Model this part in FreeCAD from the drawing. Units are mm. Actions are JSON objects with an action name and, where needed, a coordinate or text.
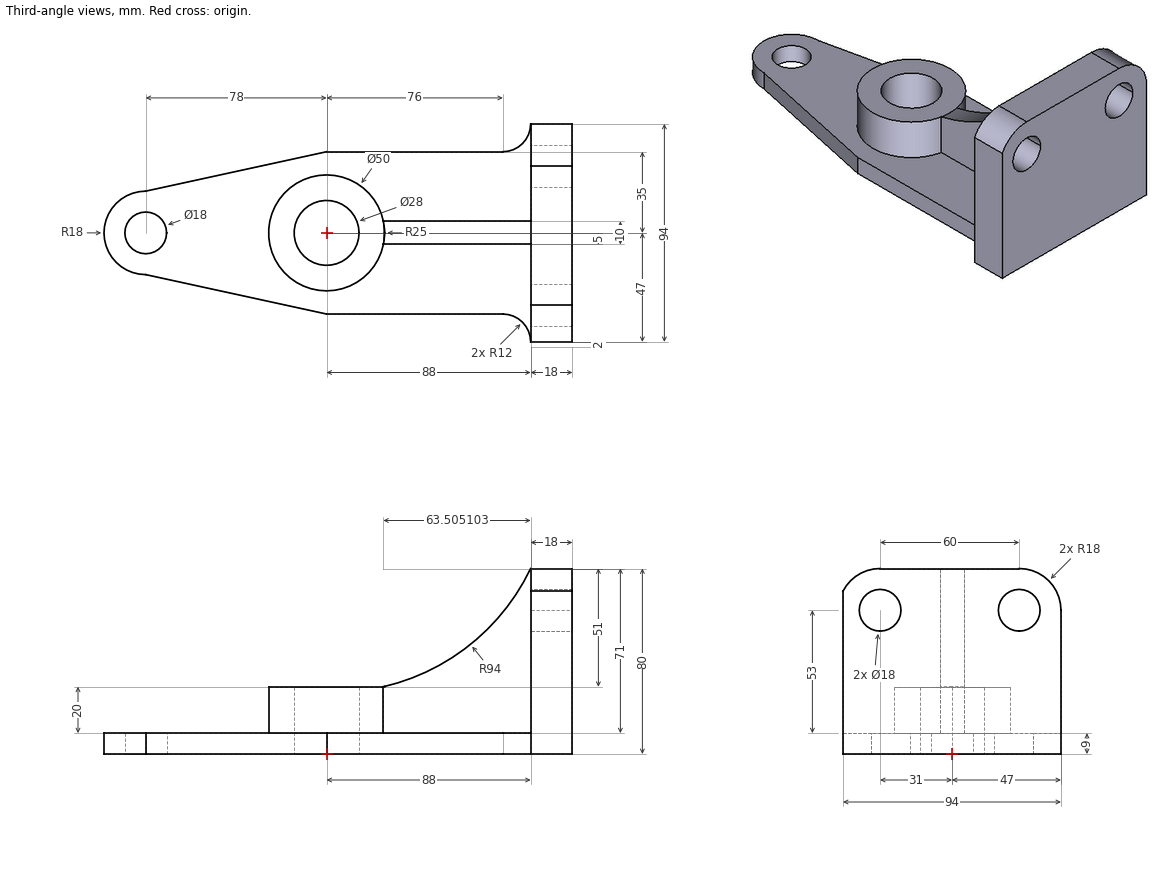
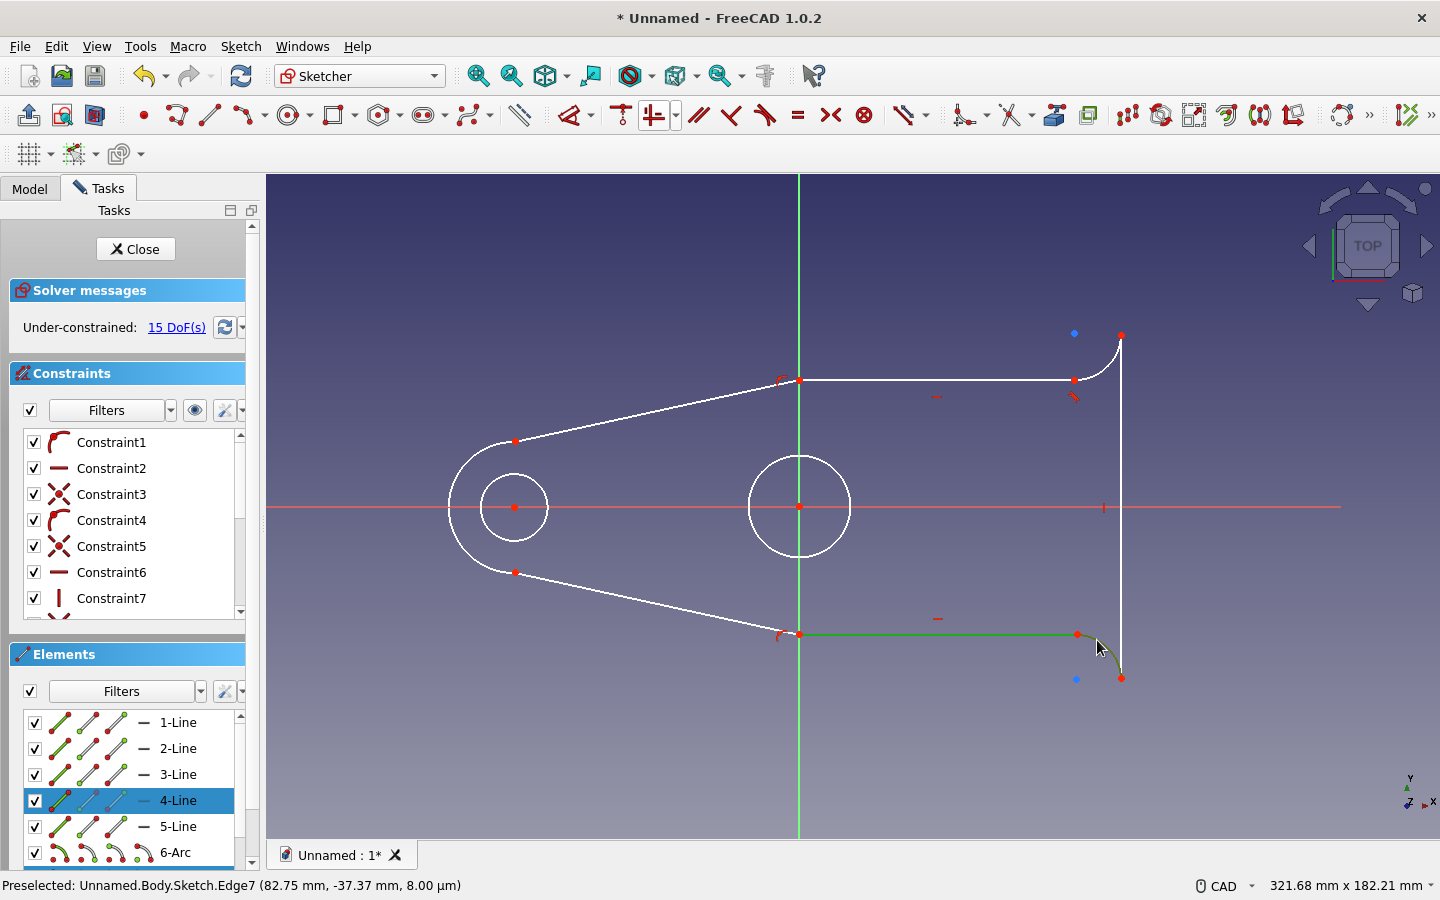
{"action": "left_click", "coordinate": [765, 116]}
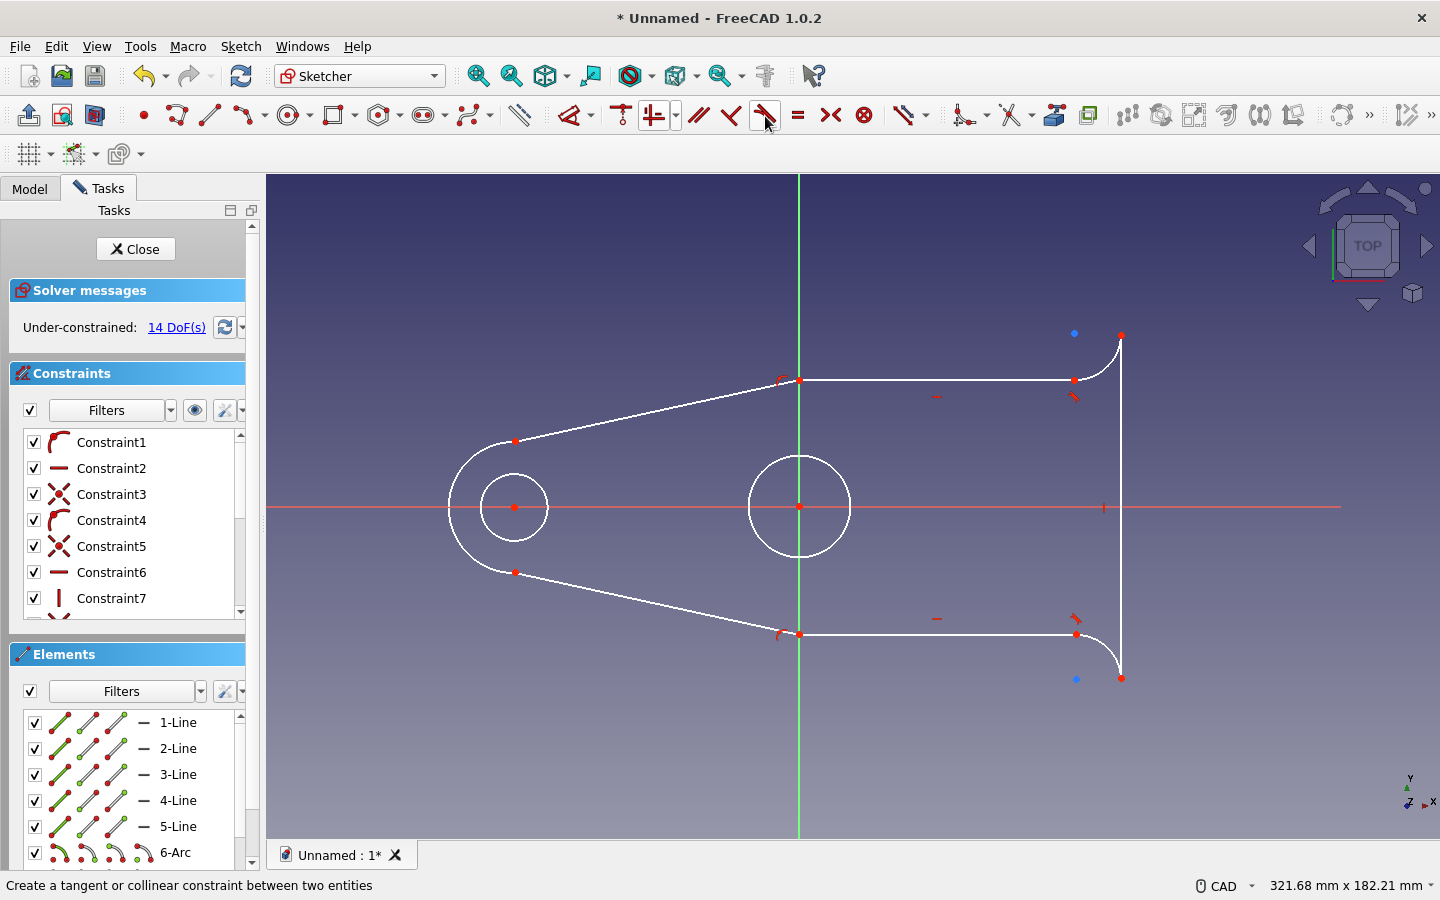
{"action": "left_click", "coordinate": [1121, 576]}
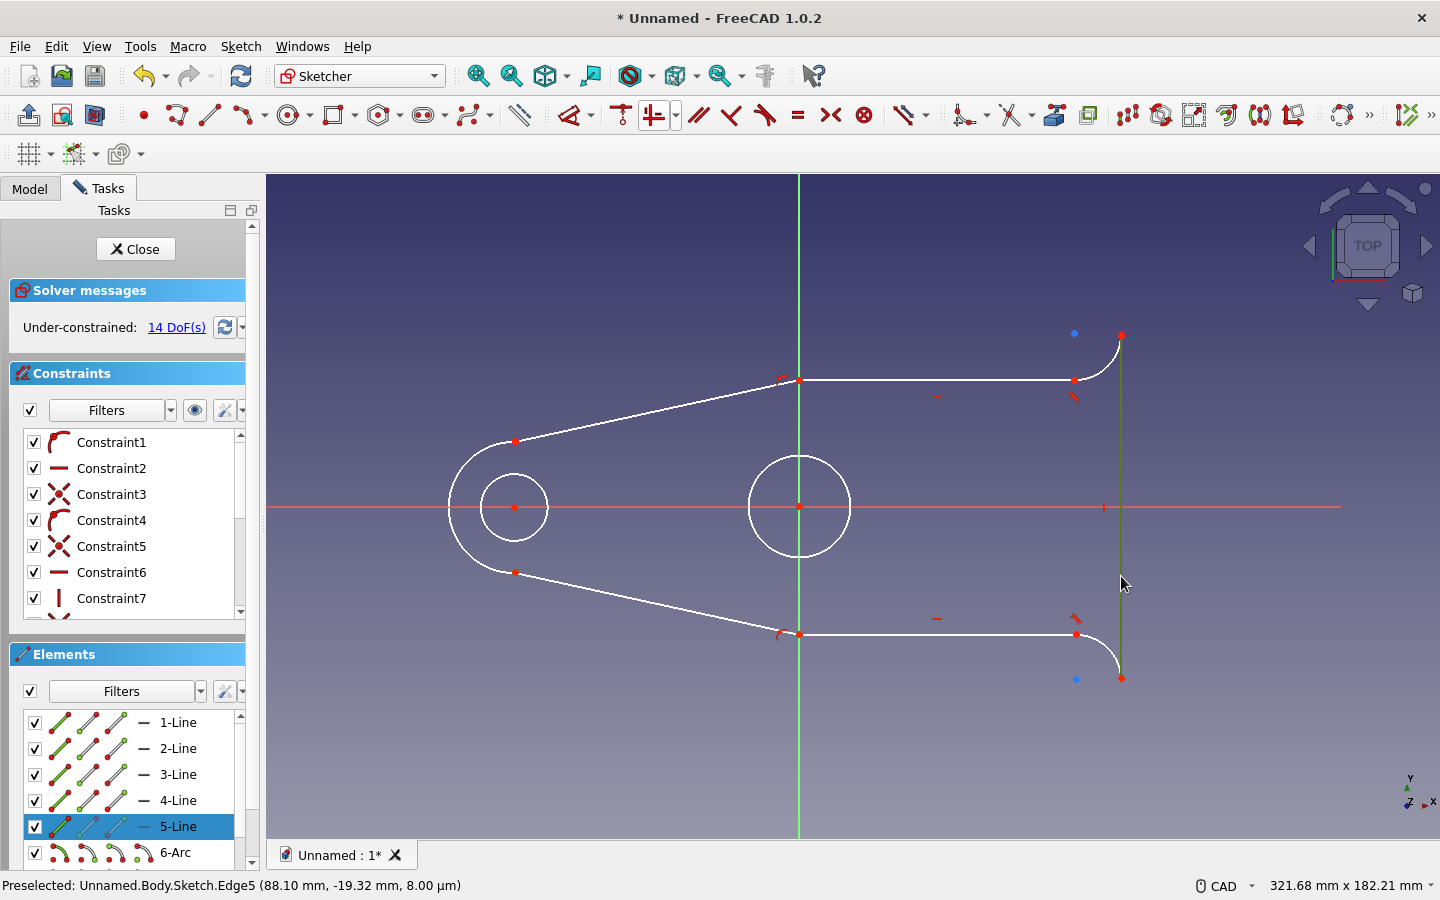
{"action": "left_click", "coordinate": [1096, 640]}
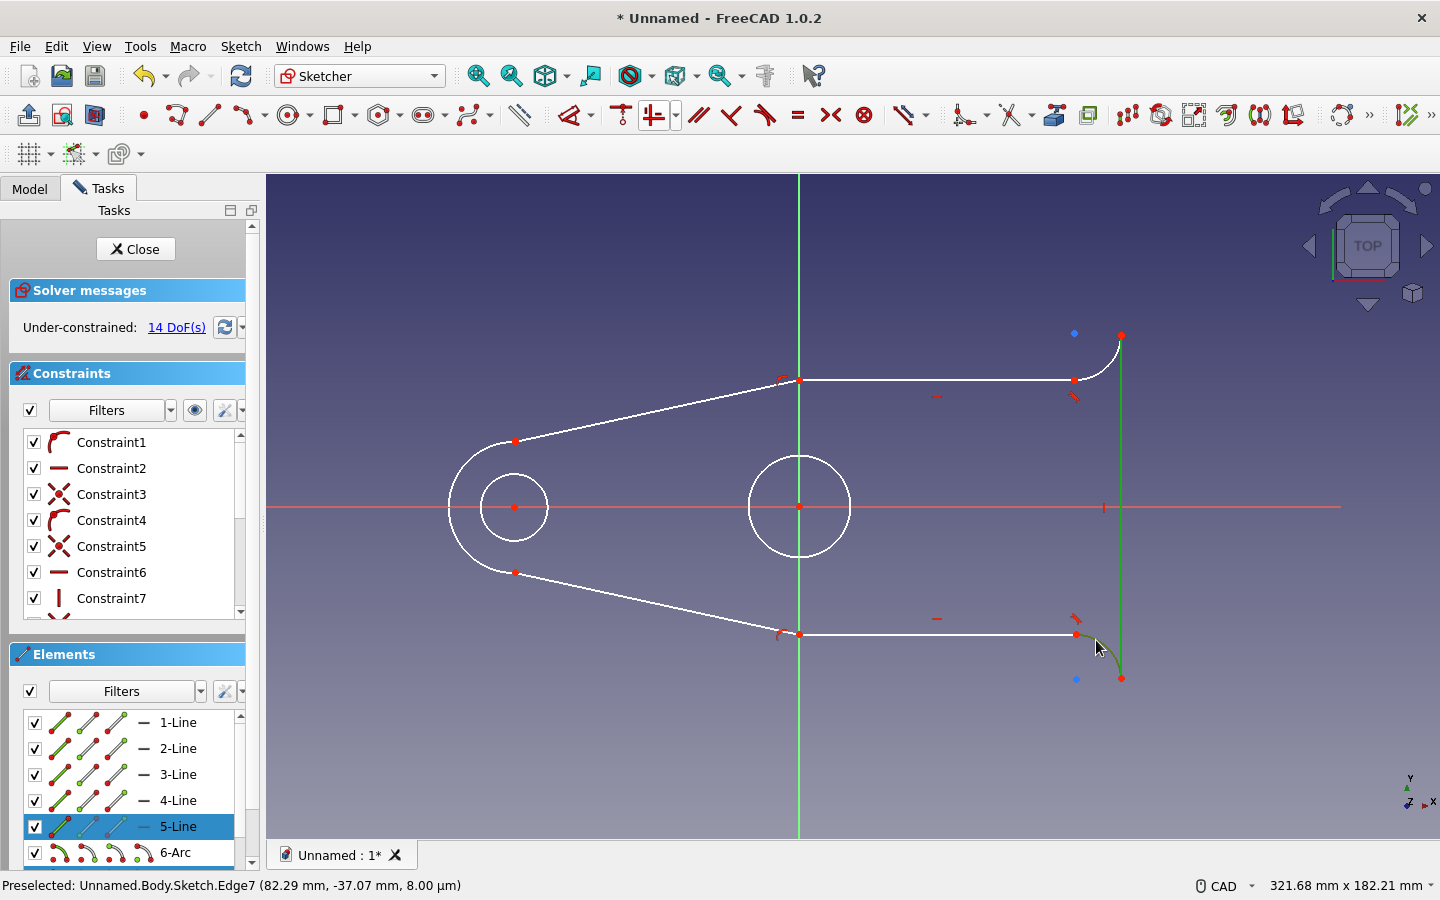
{"action": "left_click", "coordinate": [765, 116]}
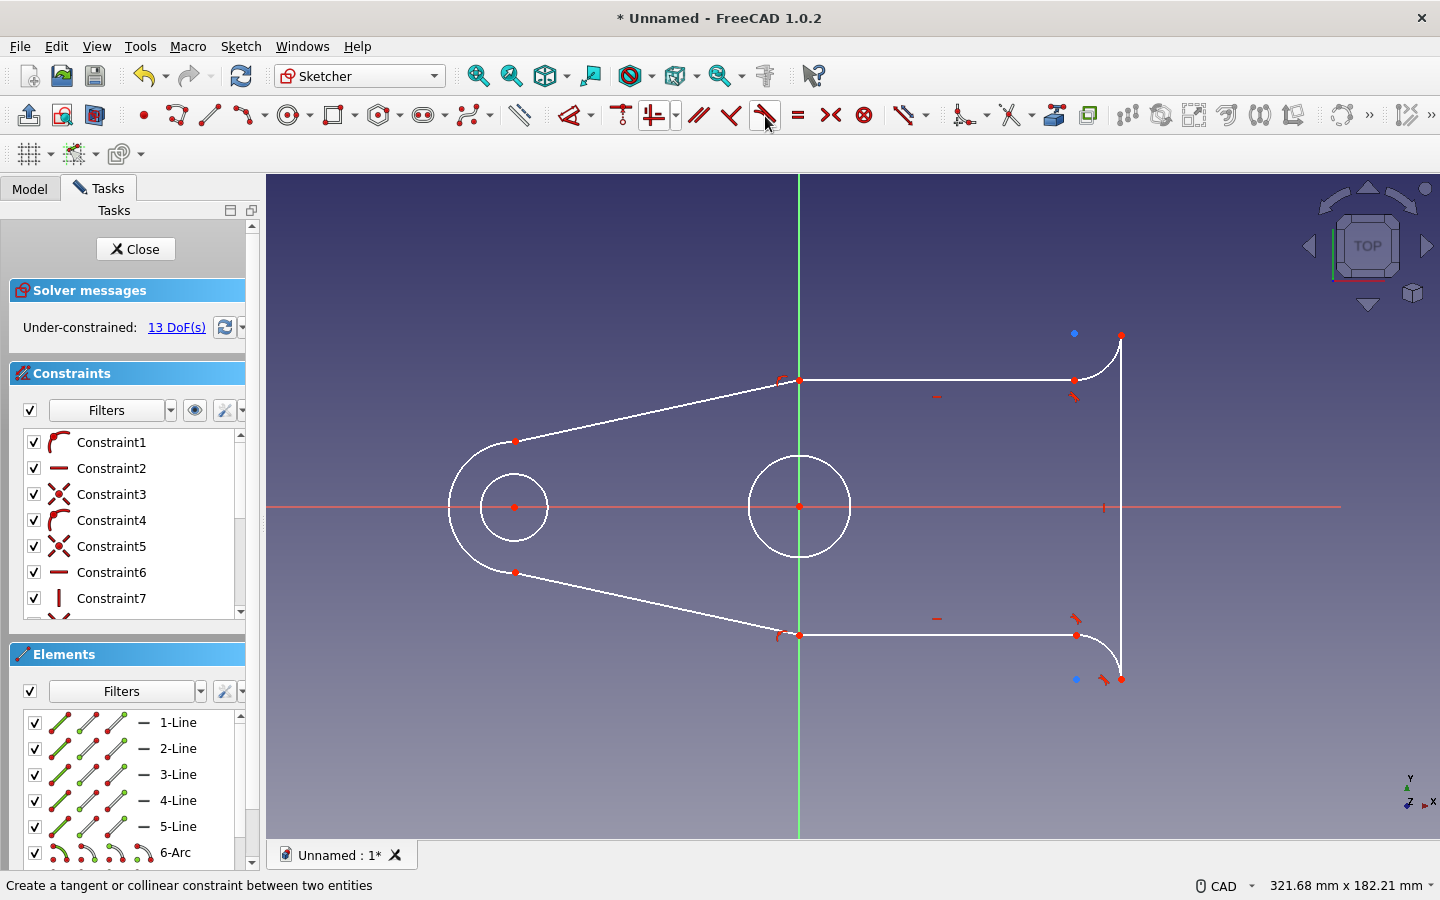
{"action": "left_click", "coordinate": [1121, 577]}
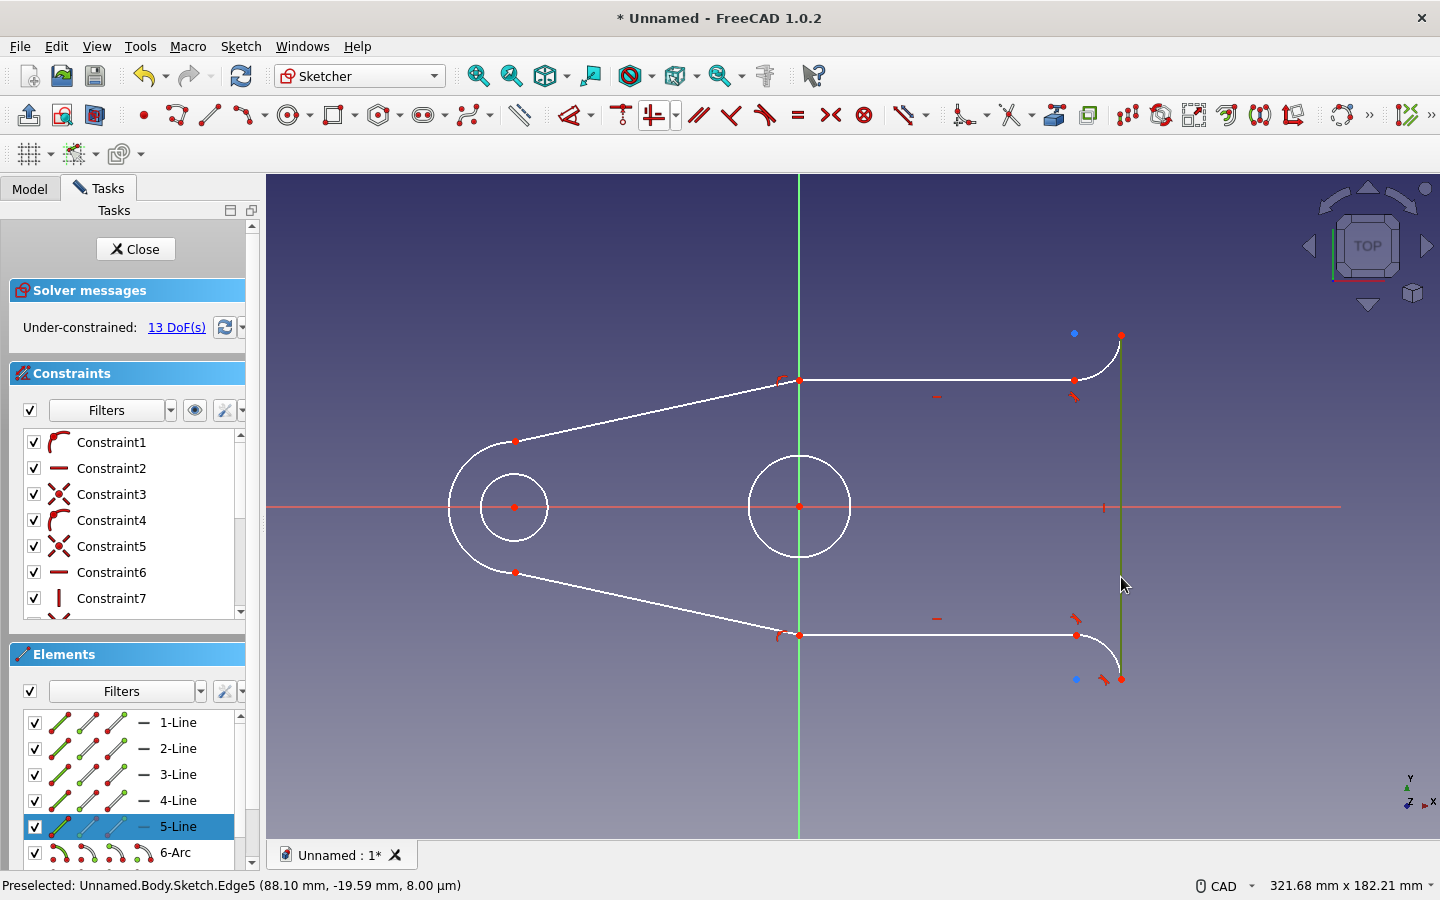
{"action": "left_click", "coordinate": [1095, 375]}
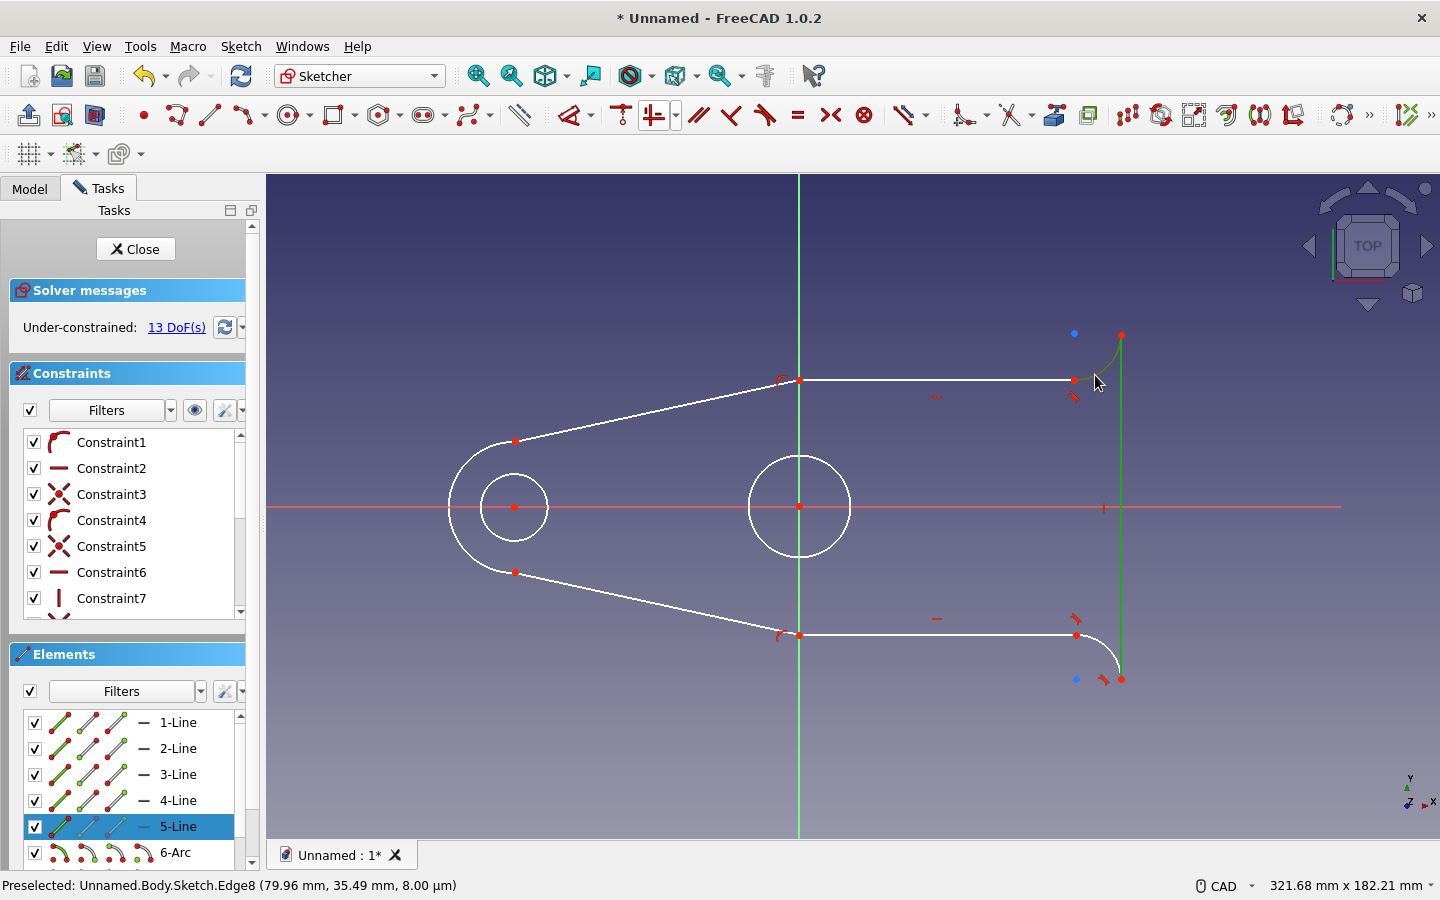
{"action": "key", "text": "t"}